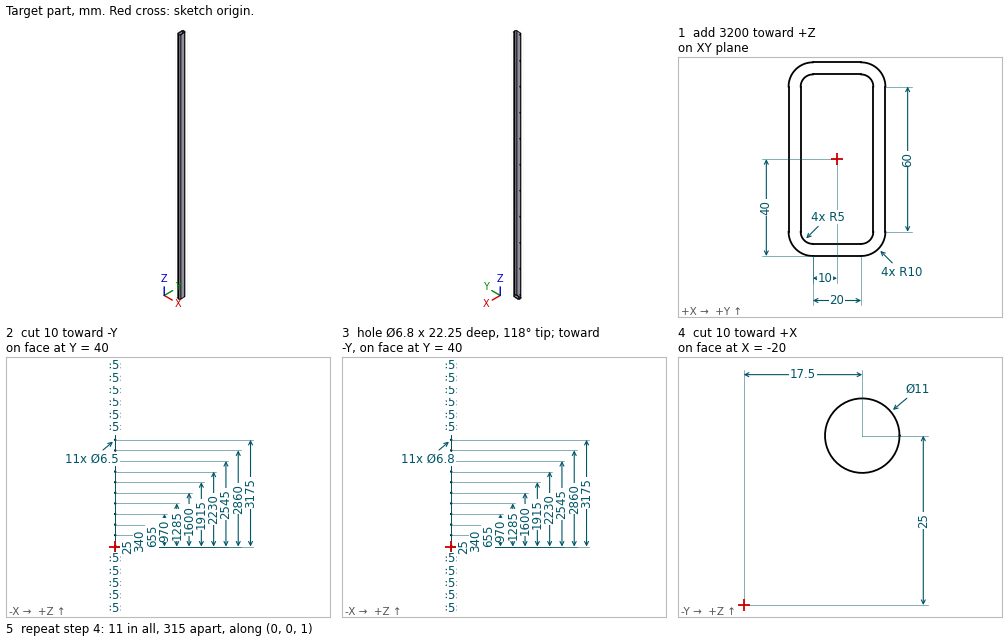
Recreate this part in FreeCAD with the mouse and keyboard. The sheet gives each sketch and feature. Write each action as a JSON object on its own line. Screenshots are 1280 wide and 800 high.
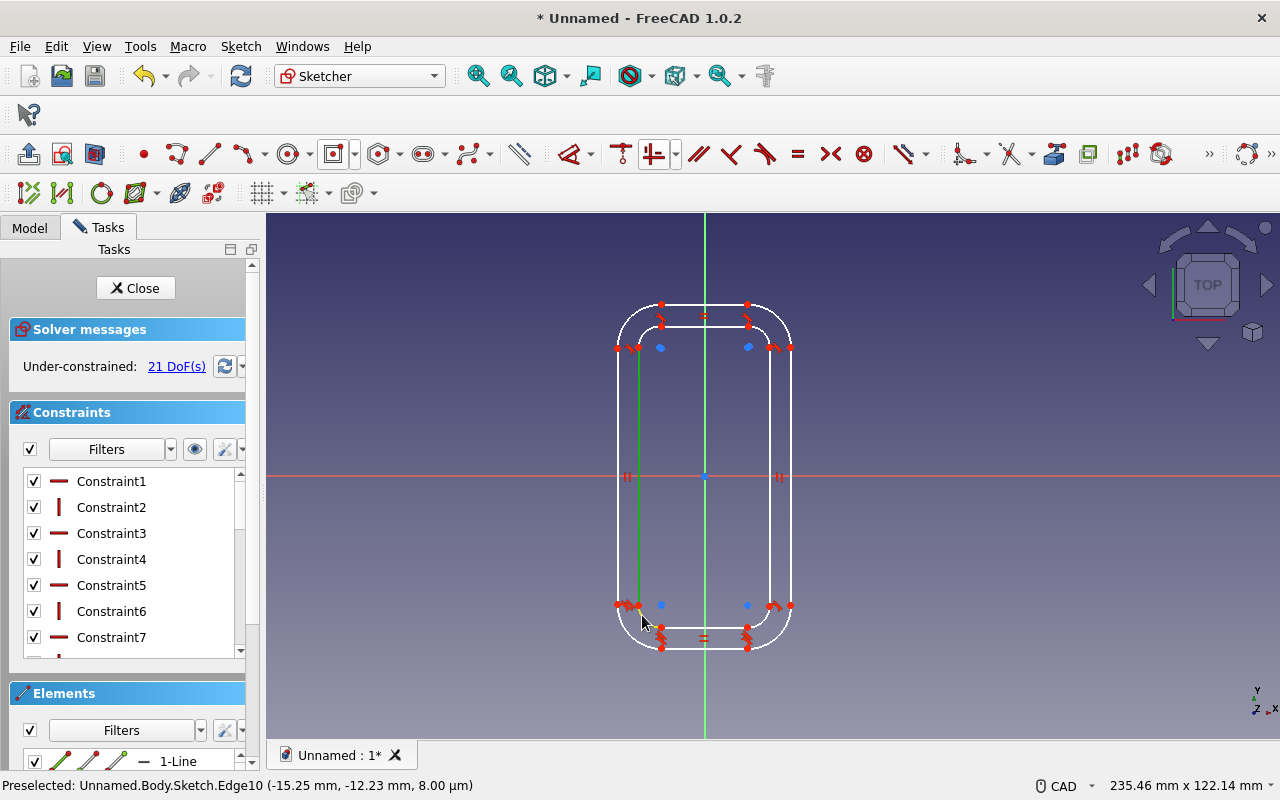
{"action": "scroll", "coordinate": [651, 328], "scroll_direction": "up", "scroll_amount": 2}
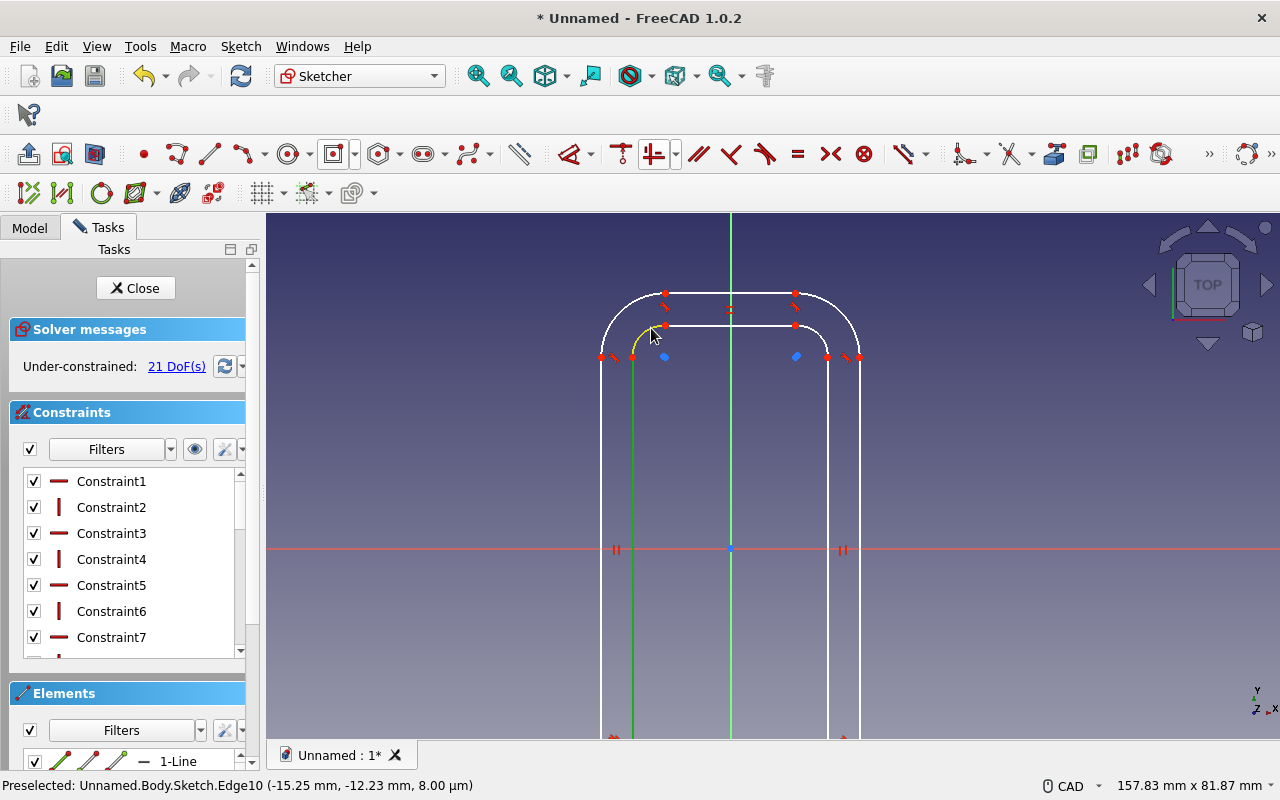
{"action": "left_click", "coordinate": [651, 328]}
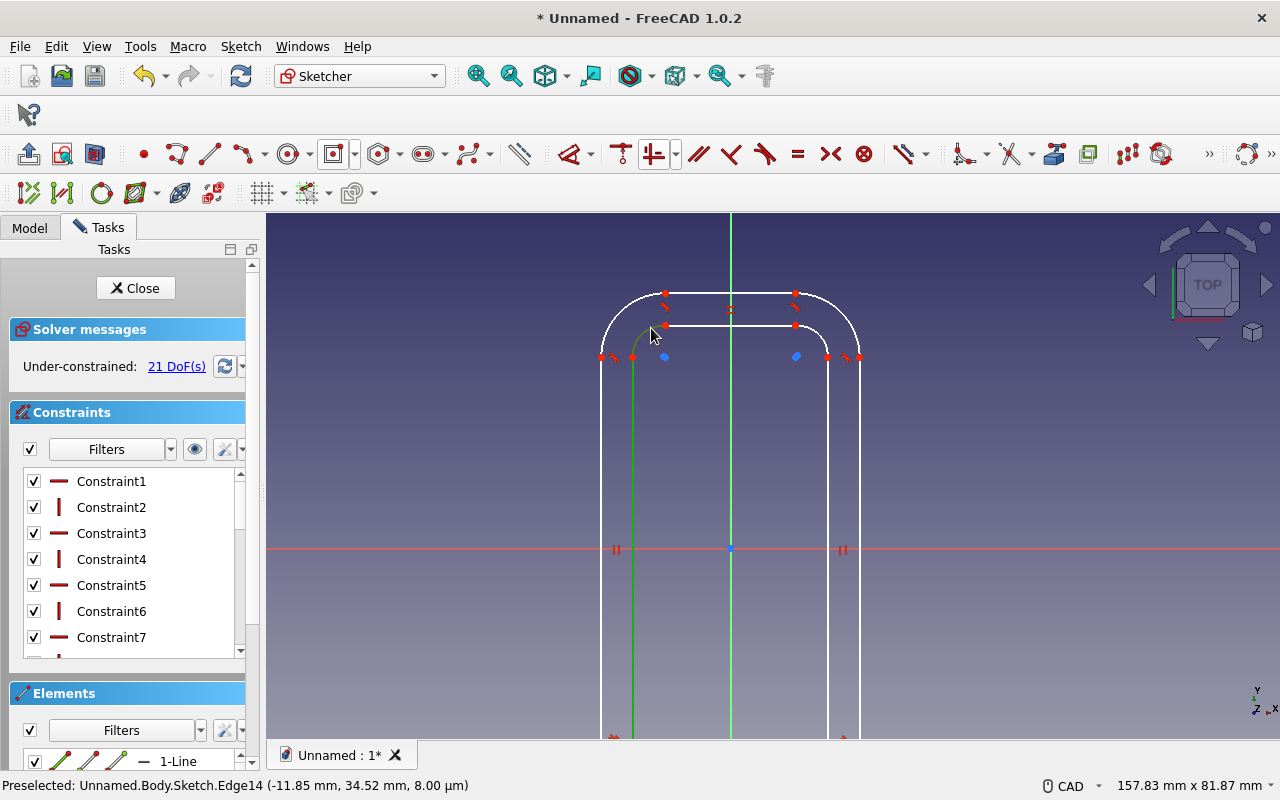
{"action": "left_click", "coordinate": [765, 154]}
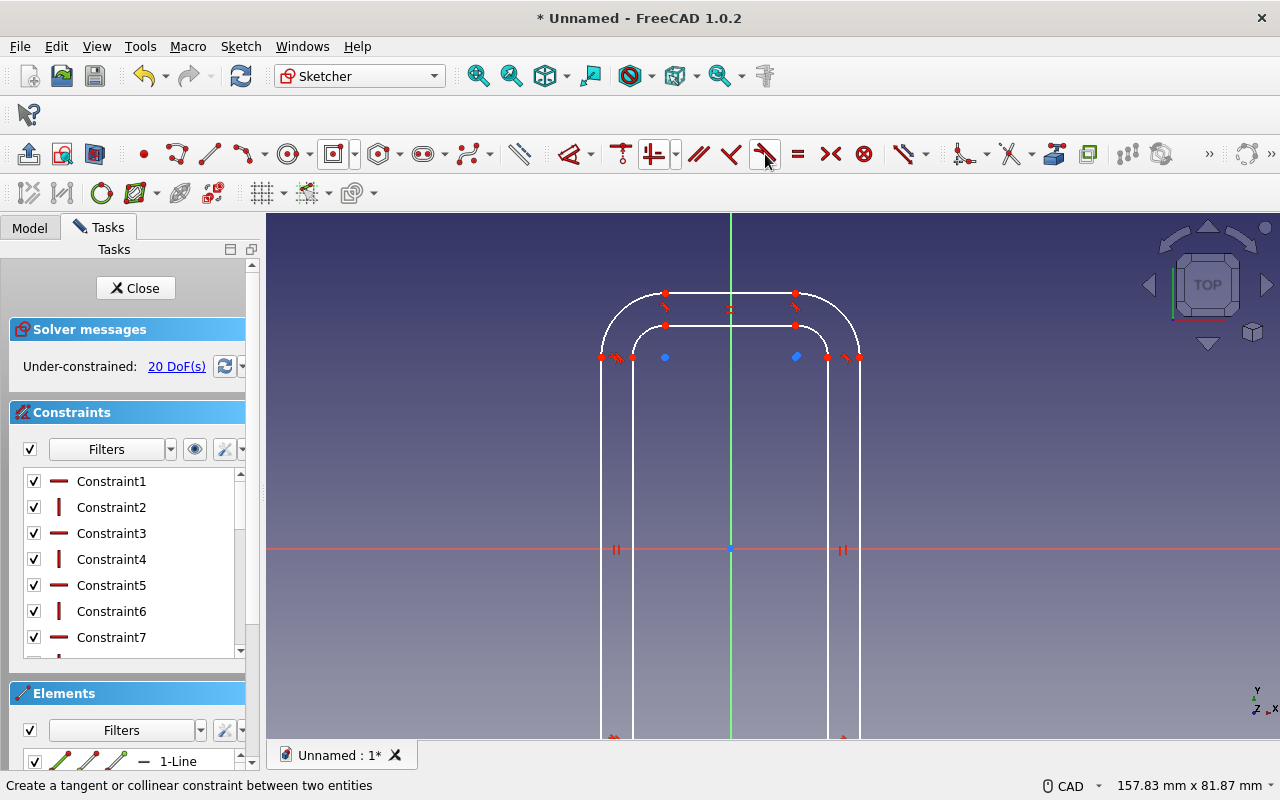
{"action": "left_click", "coordinate": [705, 326]}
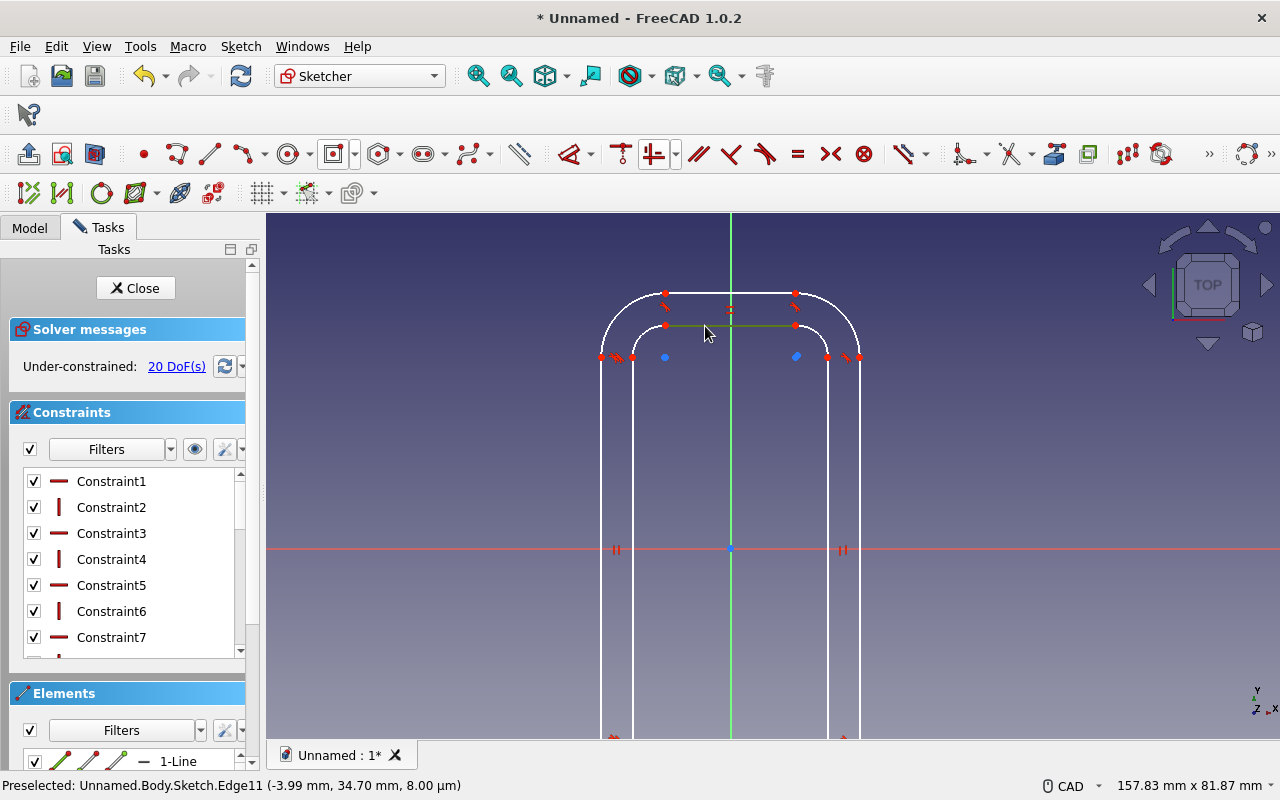
{"action": "left_click", "coordinate": [651, 329]}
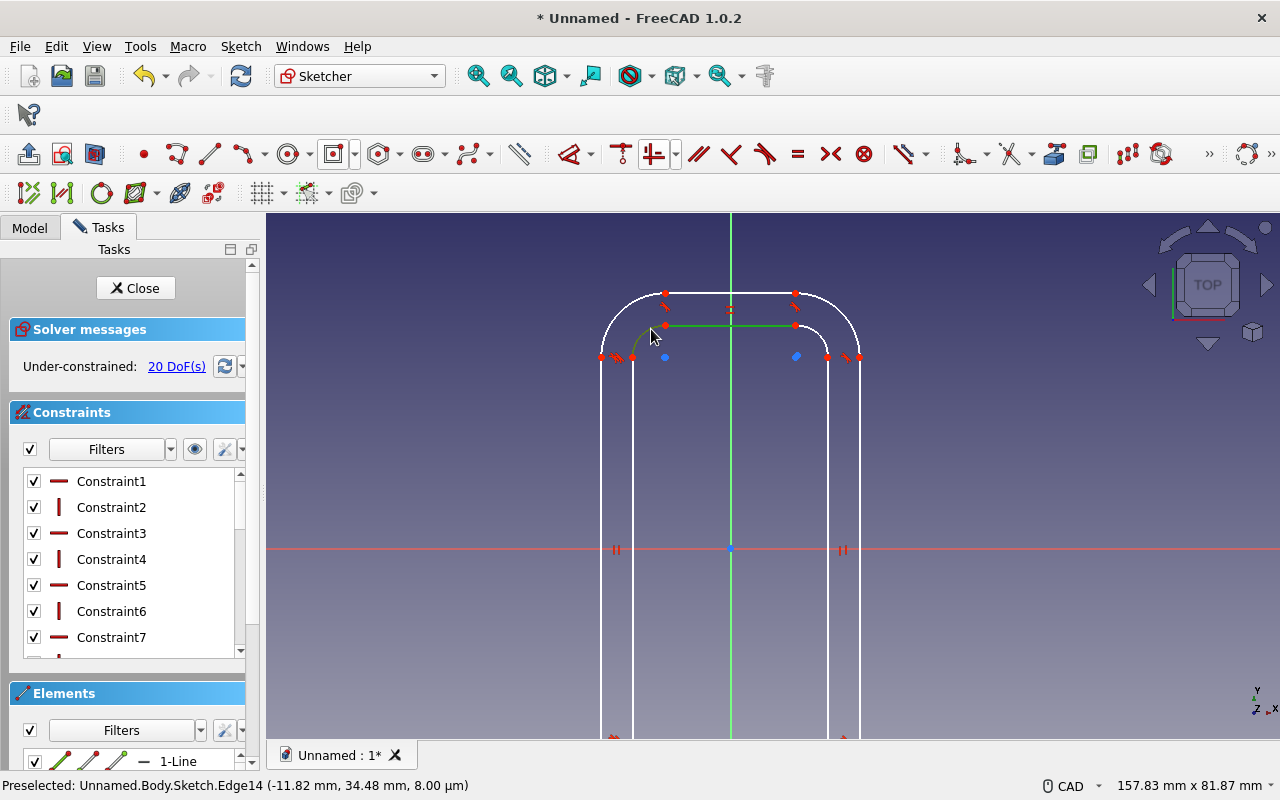
{"action": "left_click", "coordinate": [765, 154]}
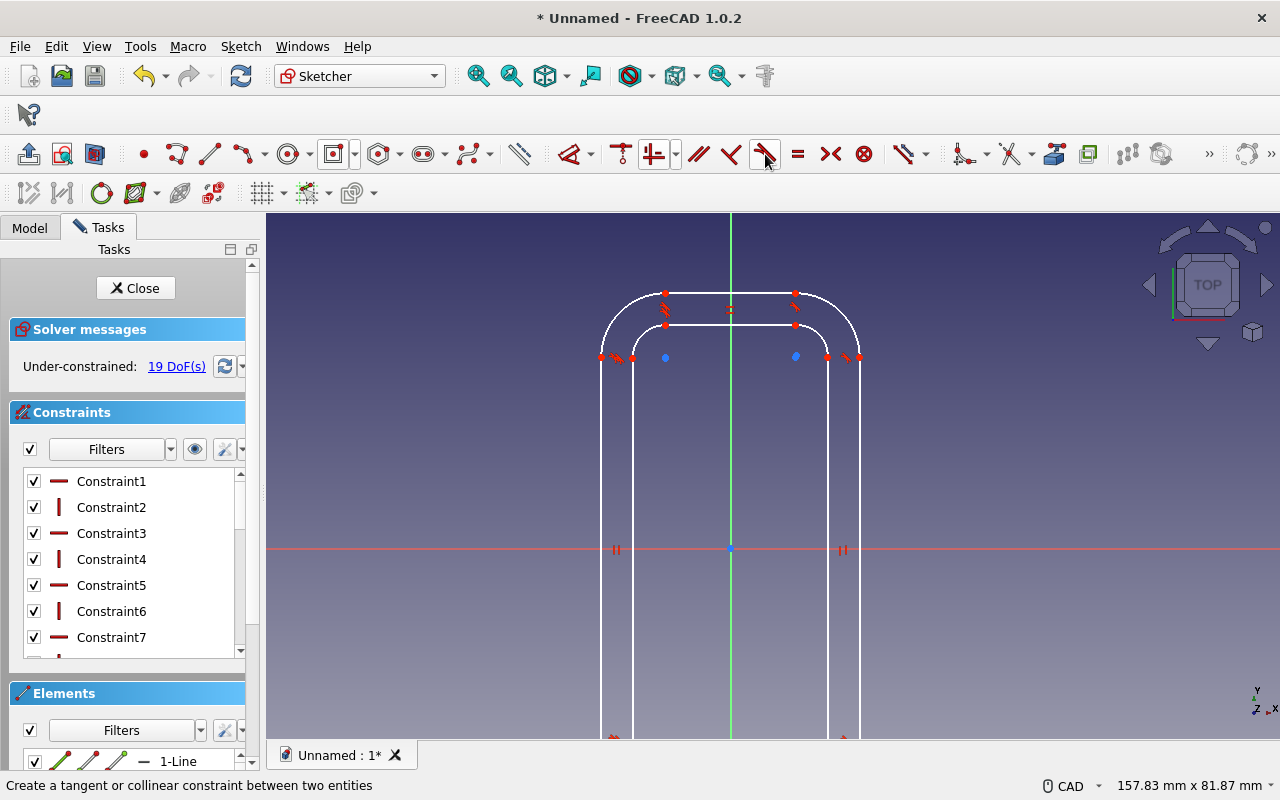
{"action": "left_click", "coordinate": [705, 325]}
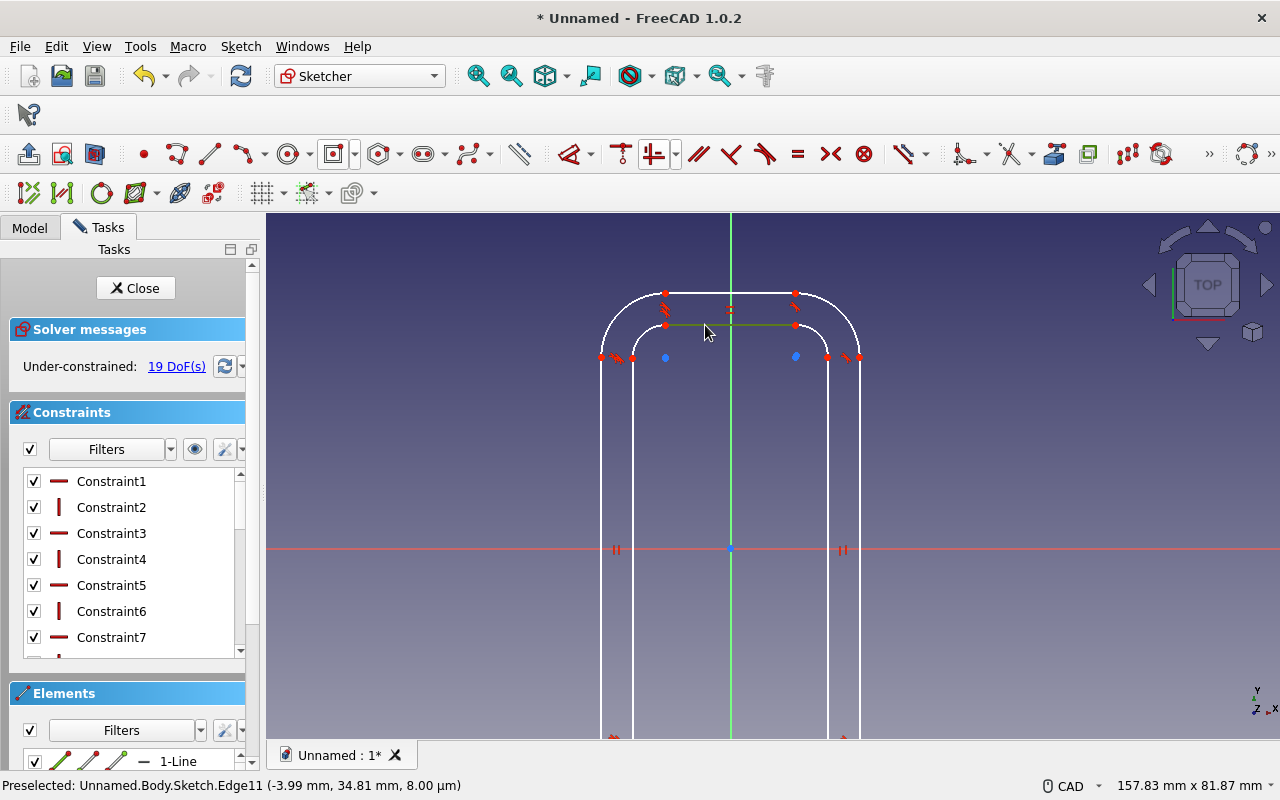
{"action": "left_click", "coordinate": [825, 342]}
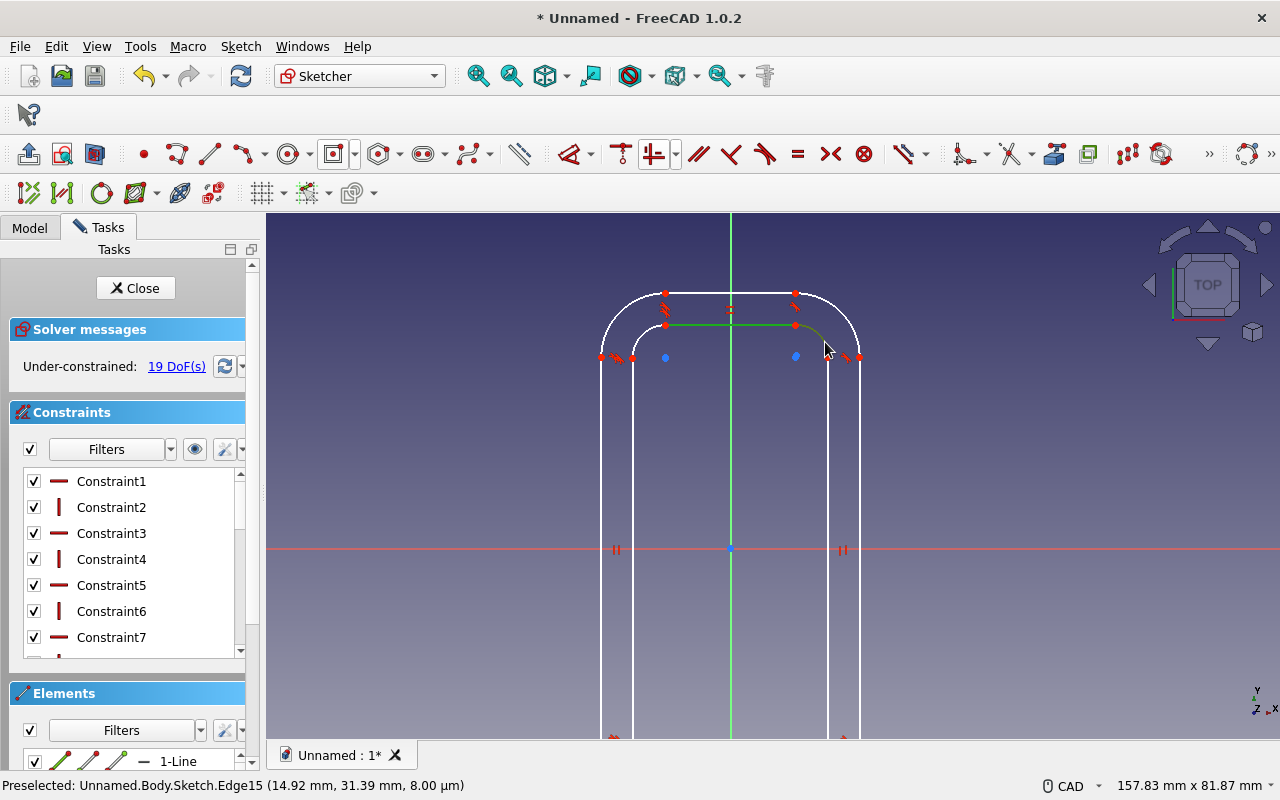
{"action": "left_click", "coordinate": [765, 154]}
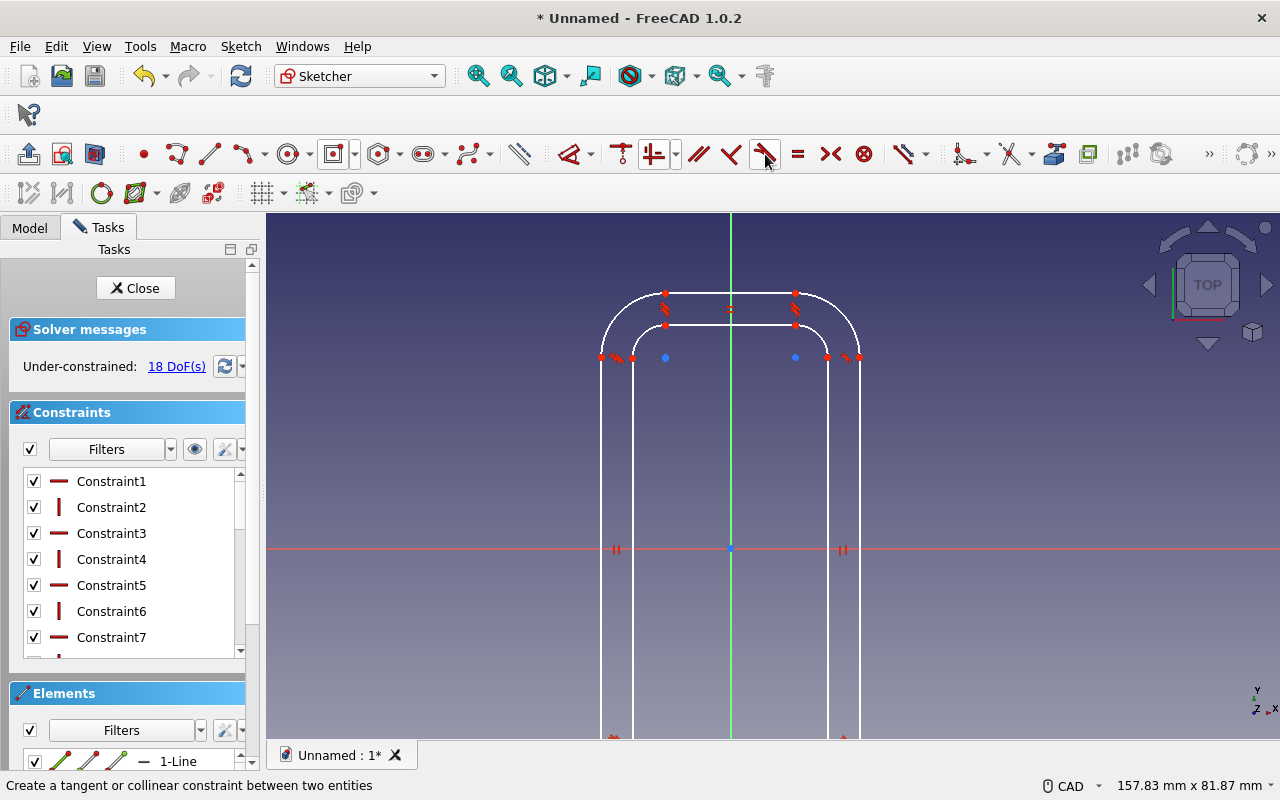
{"action": "left_click", "coordinate": [828, 473]}